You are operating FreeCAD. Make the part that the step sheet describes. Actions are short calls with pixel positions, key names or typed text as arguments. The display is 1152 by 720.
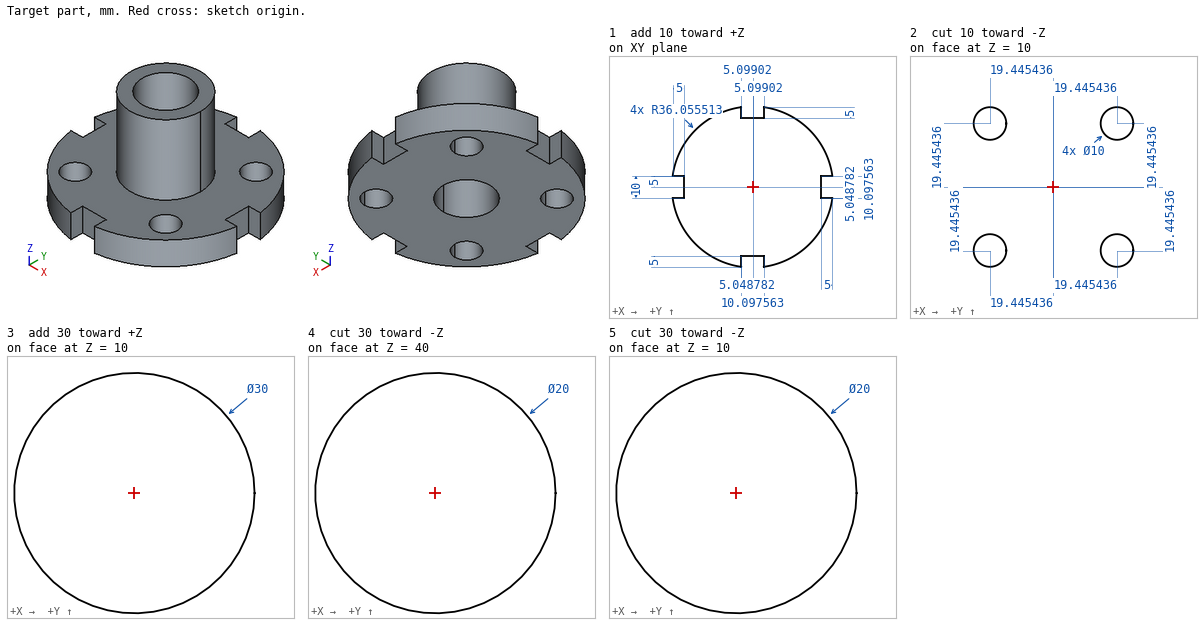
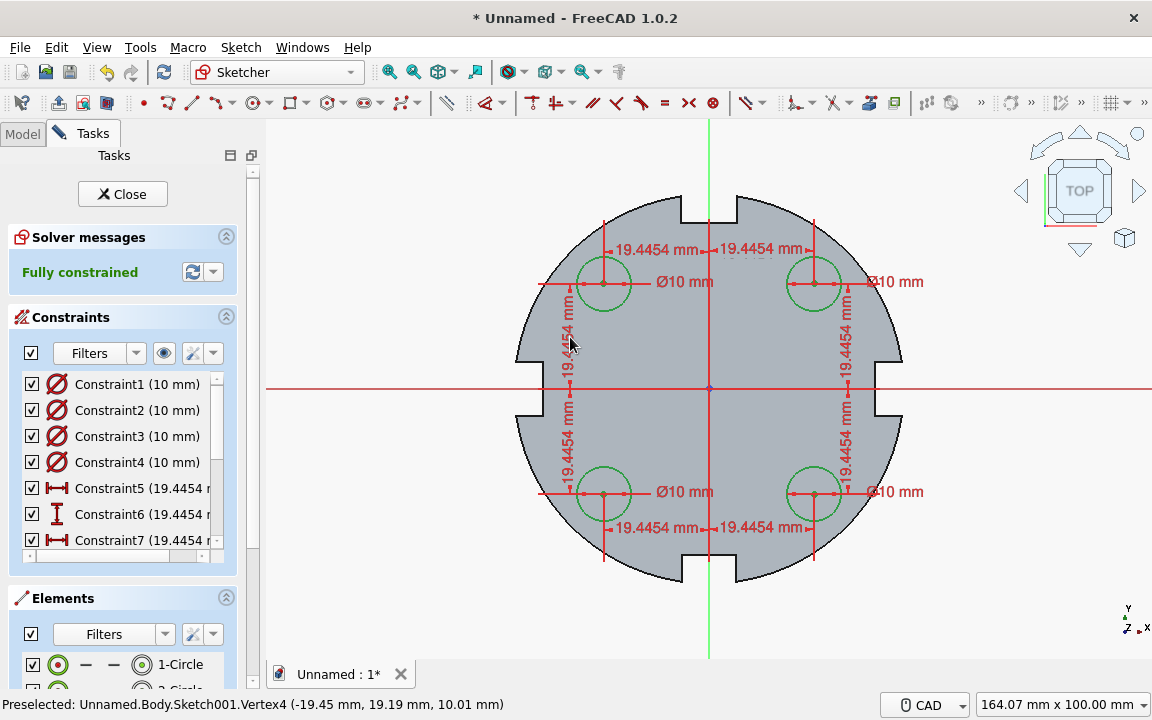
click(123, 194)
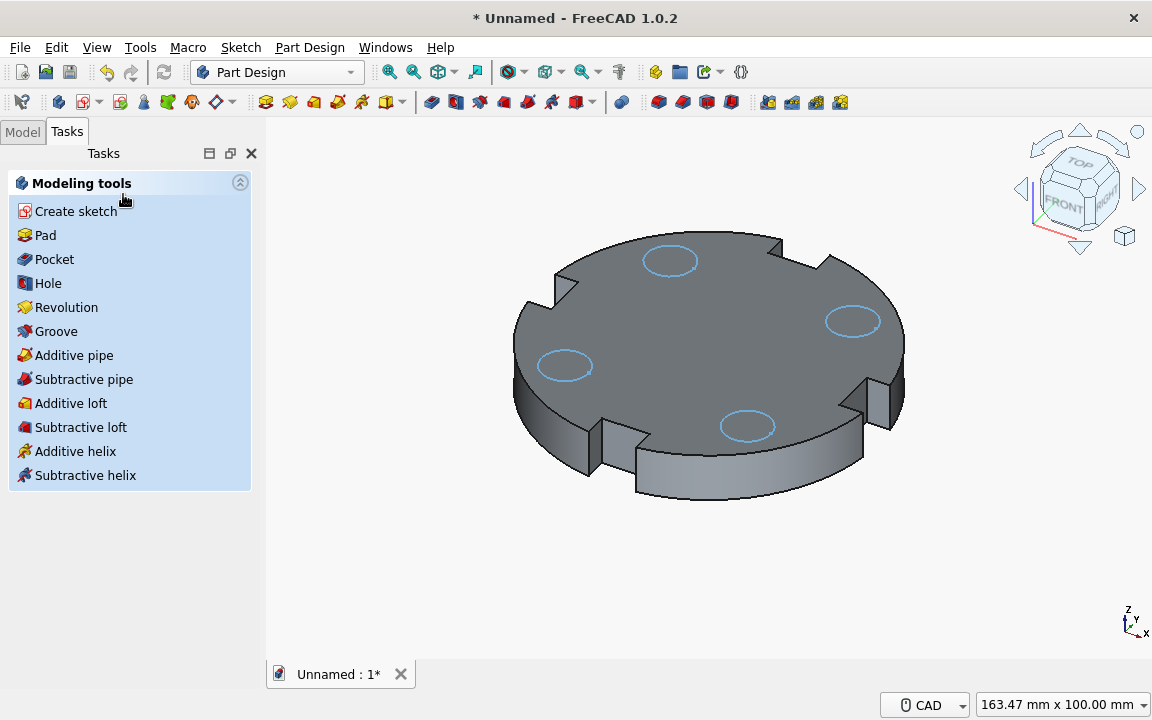
click(432, 102)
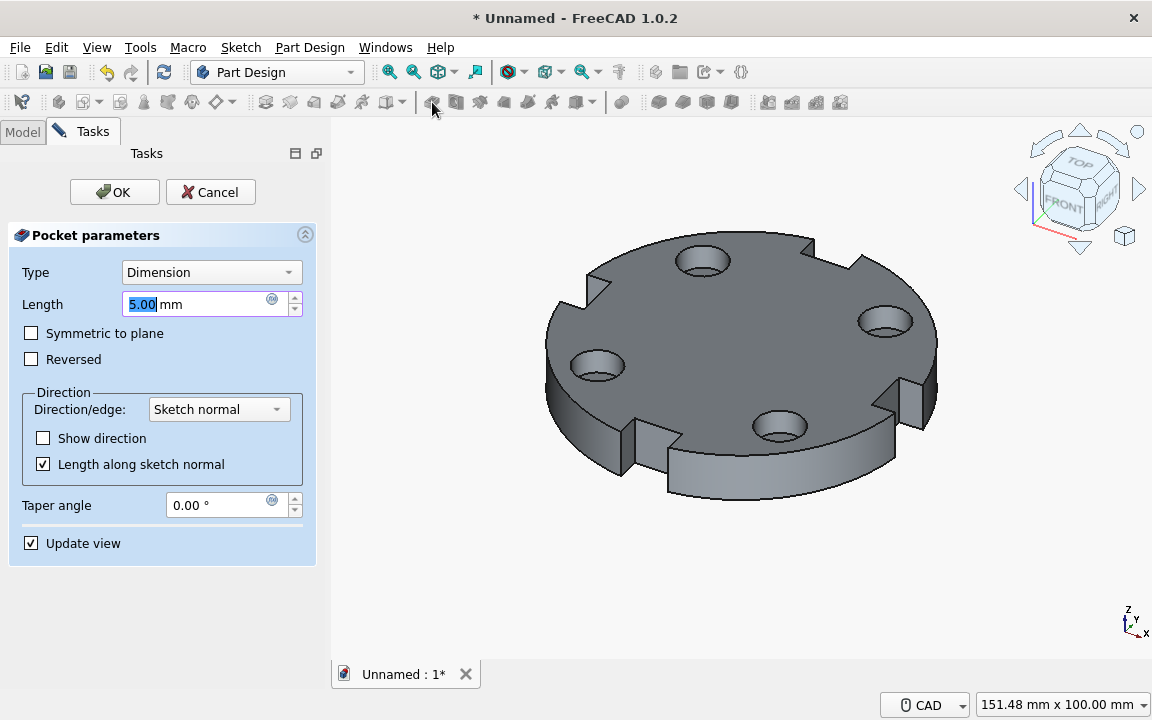
text(10)
key(Tab)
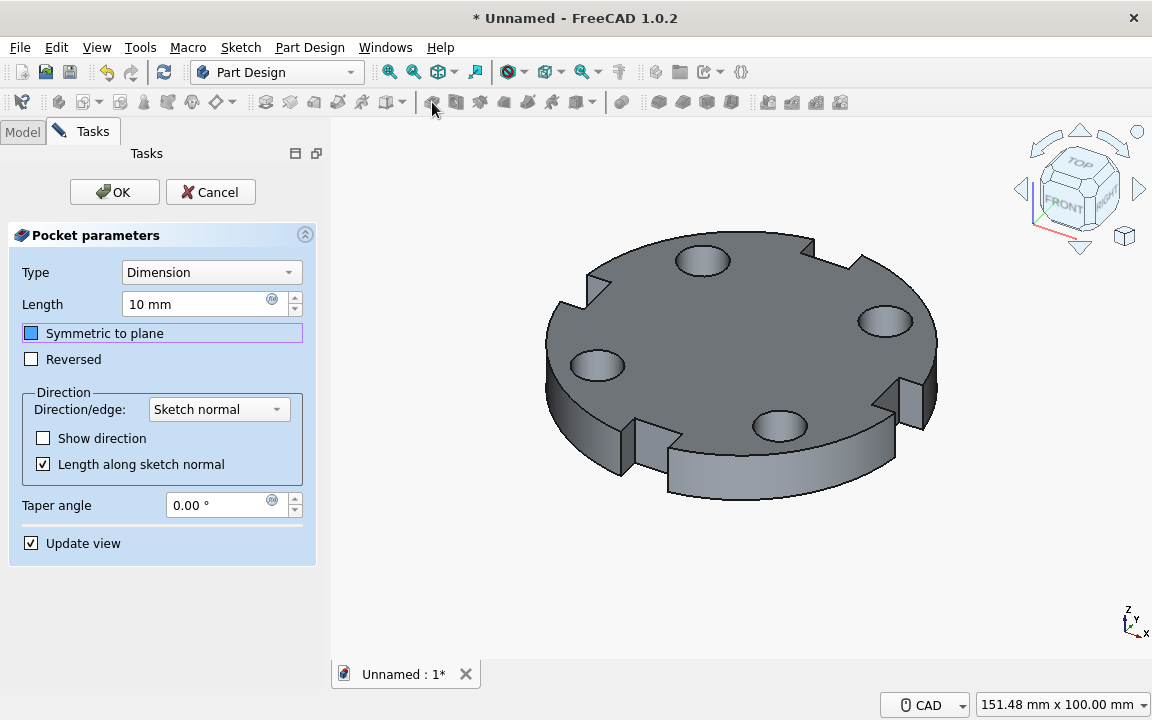
click(115, 192)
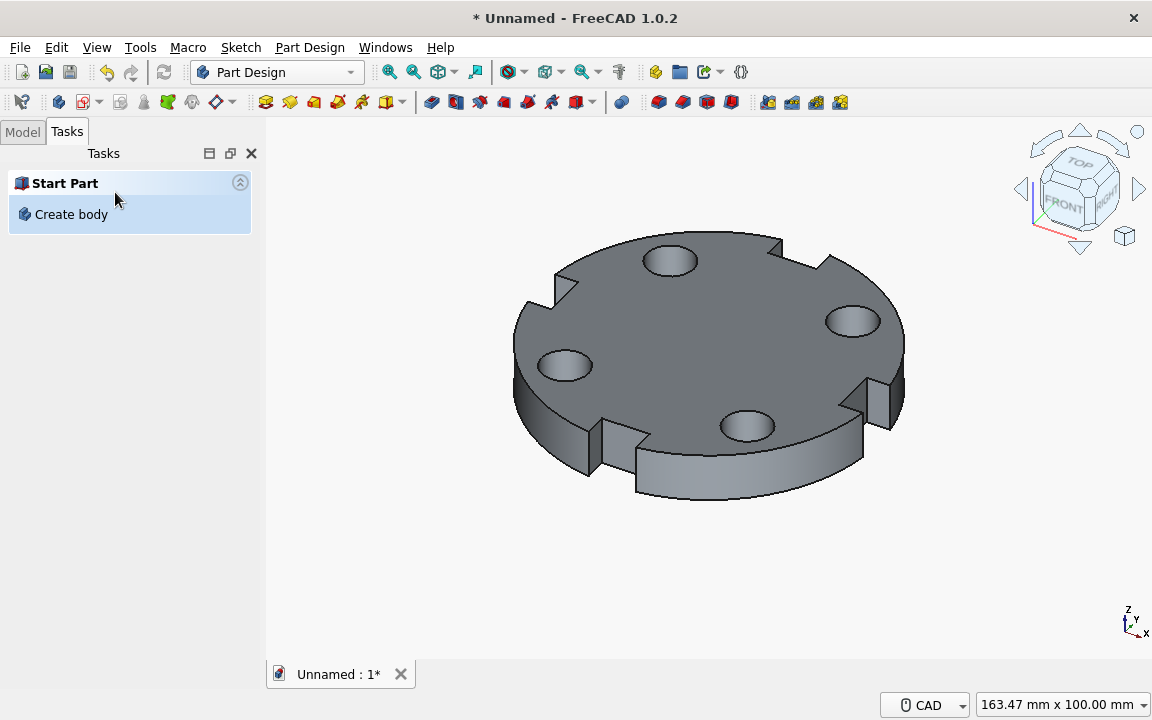
click(709, 343)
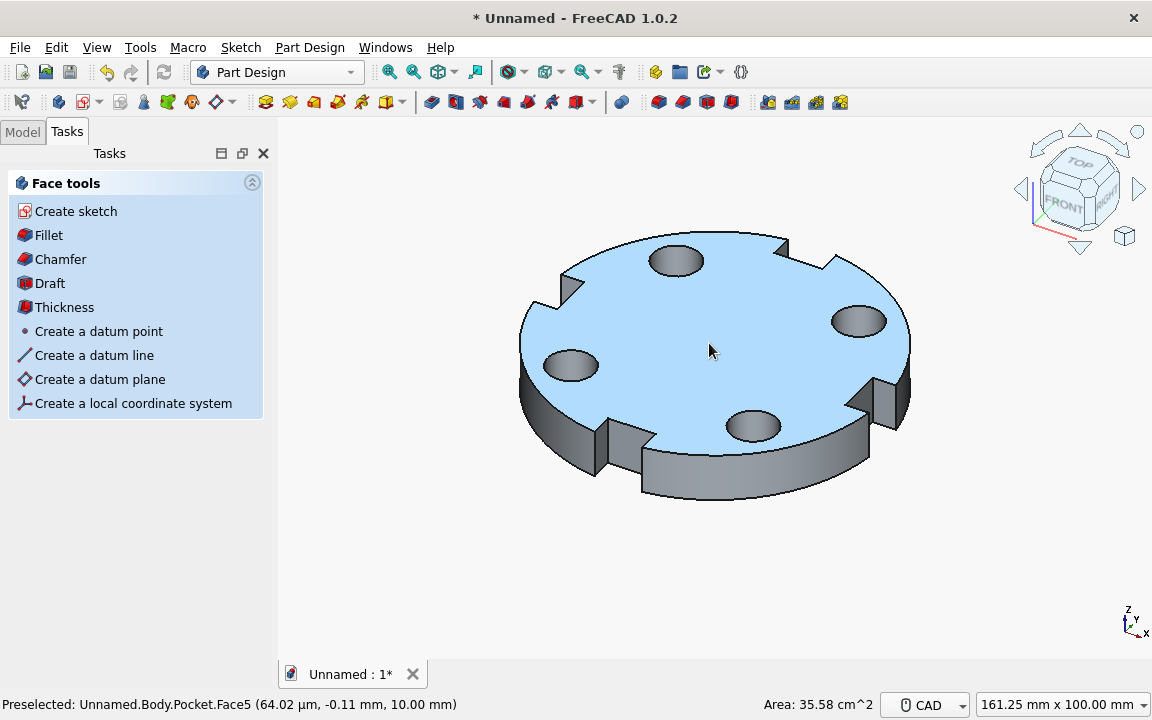
click(84, 102)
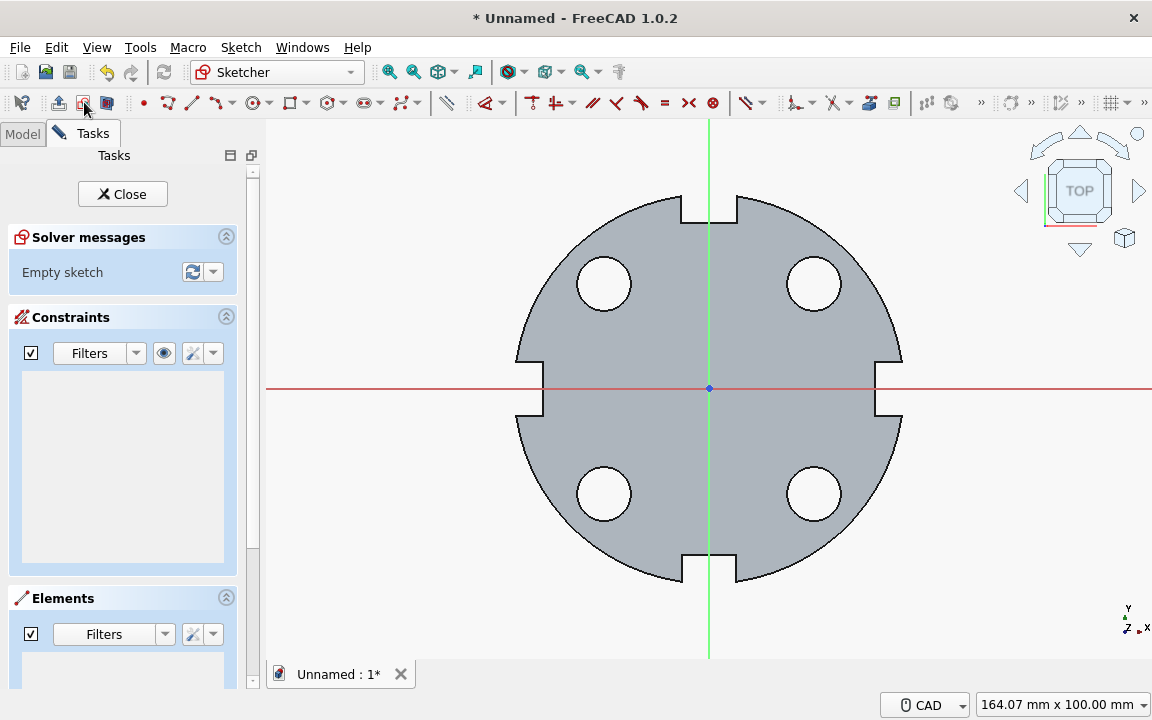
scroll(765, 389, up, 4)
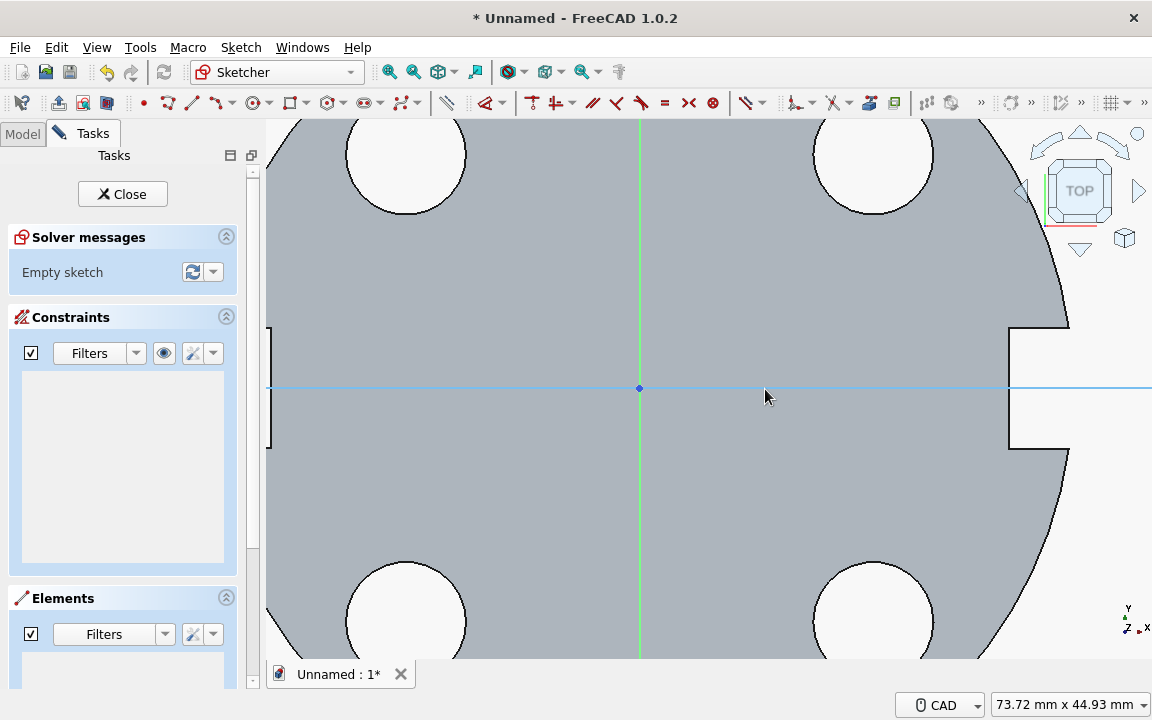
click(254, 104)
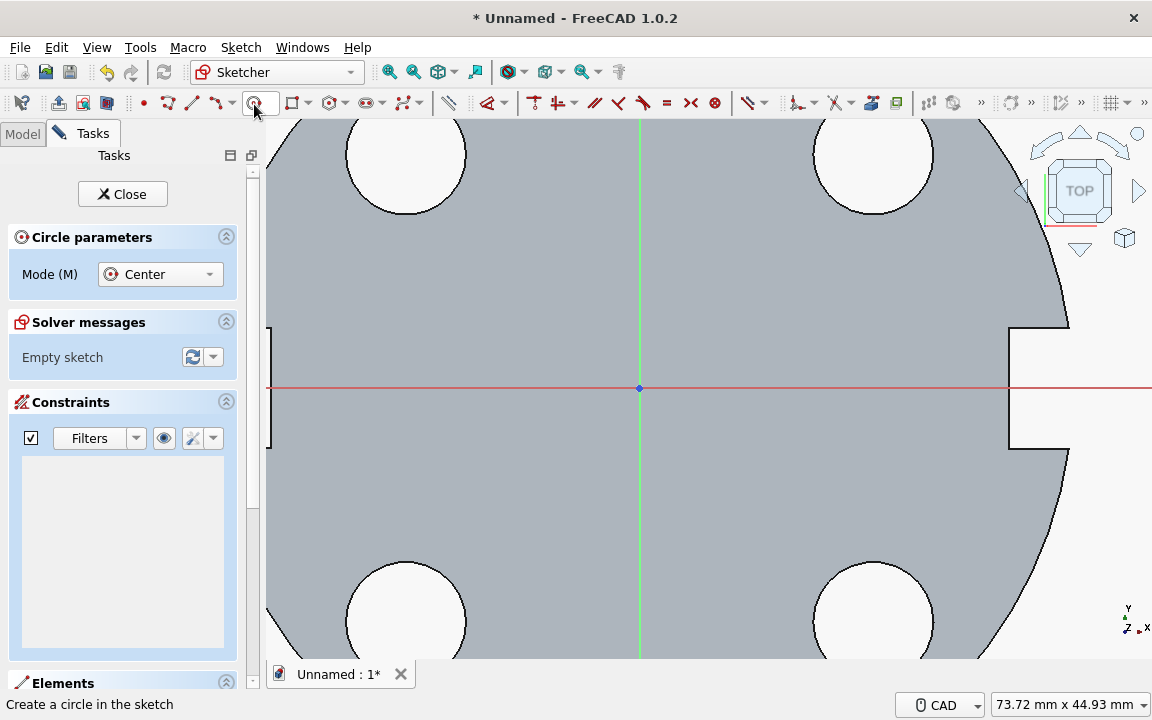
click(640, 388)
move(767, 261)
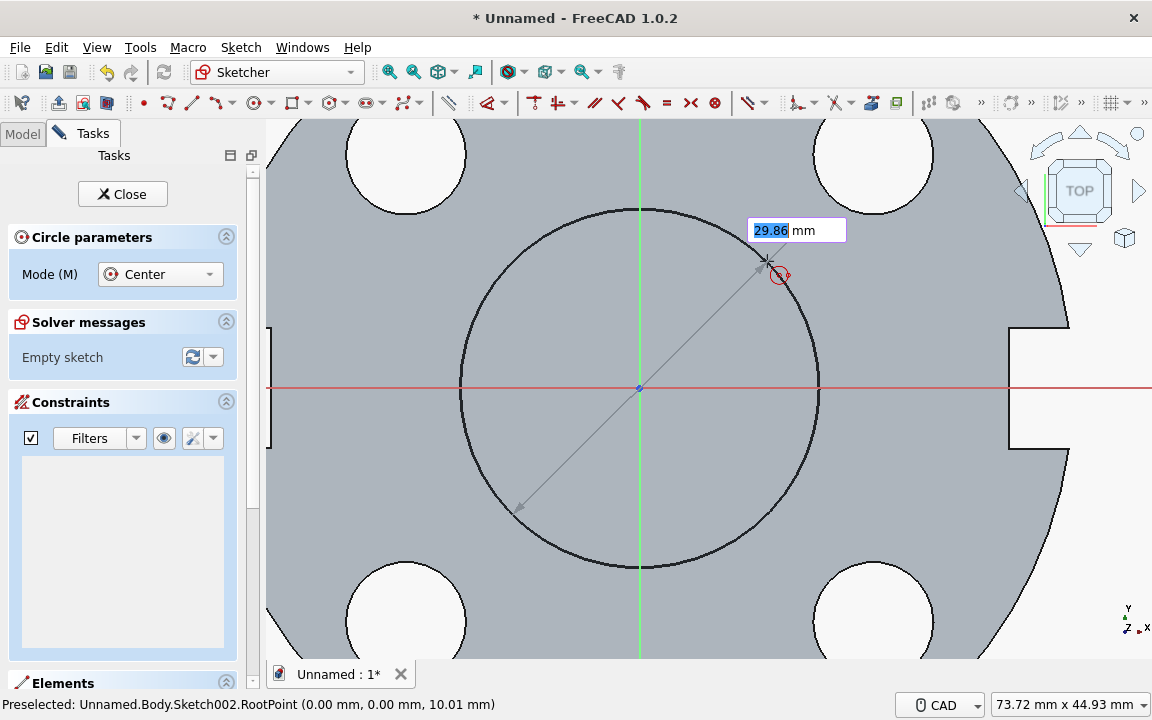
text(30)
key(Return)
key(Escape)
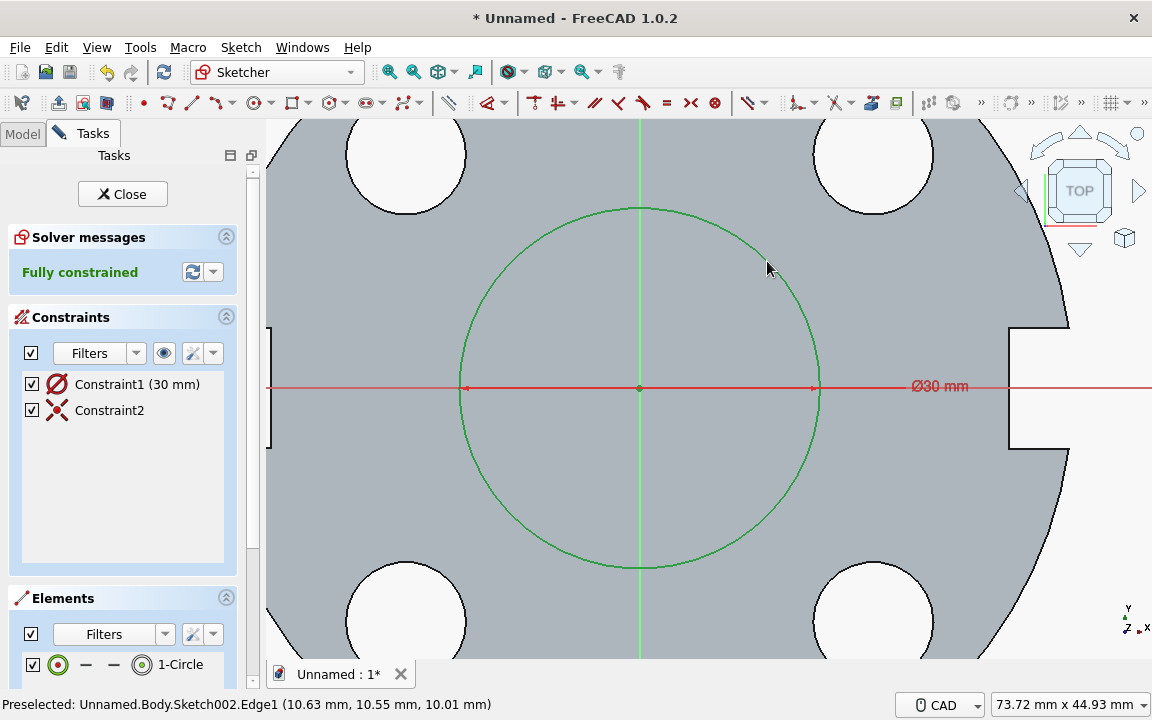
click(123, 194)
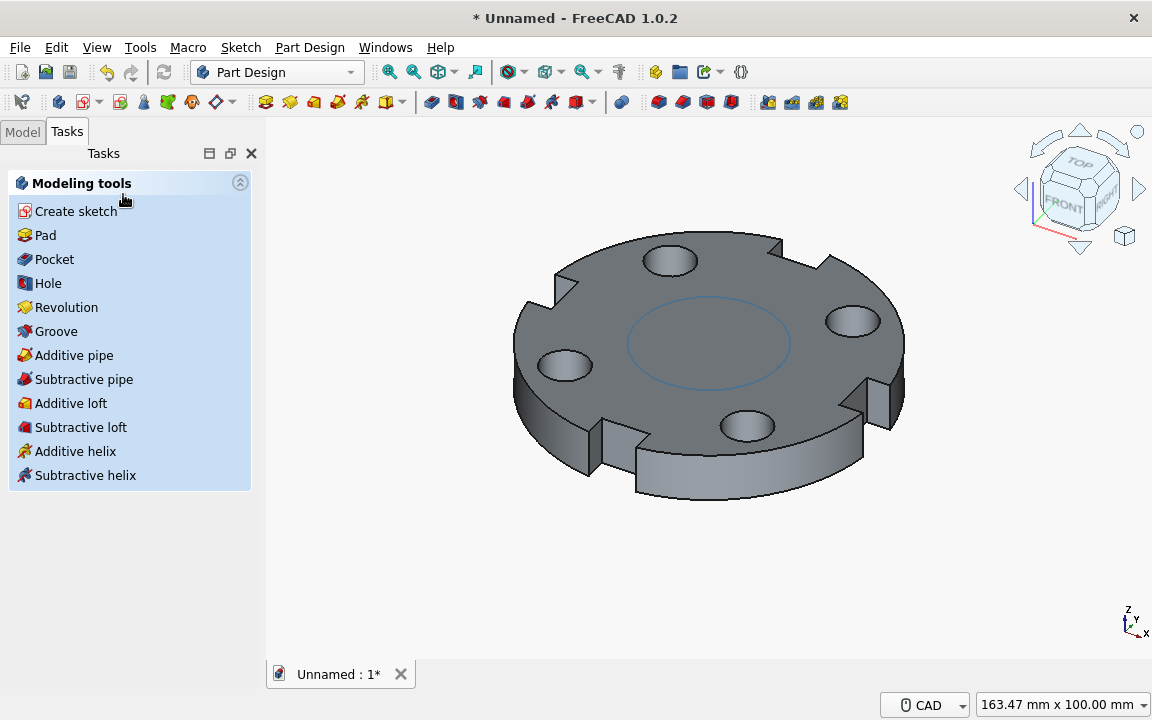
click(266, 102)